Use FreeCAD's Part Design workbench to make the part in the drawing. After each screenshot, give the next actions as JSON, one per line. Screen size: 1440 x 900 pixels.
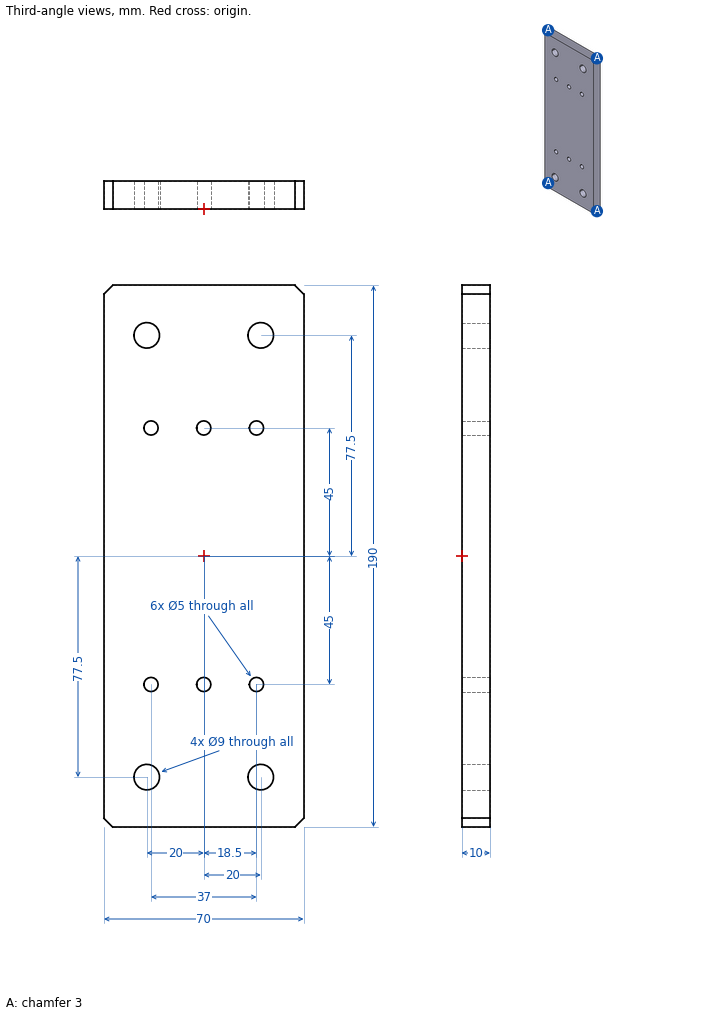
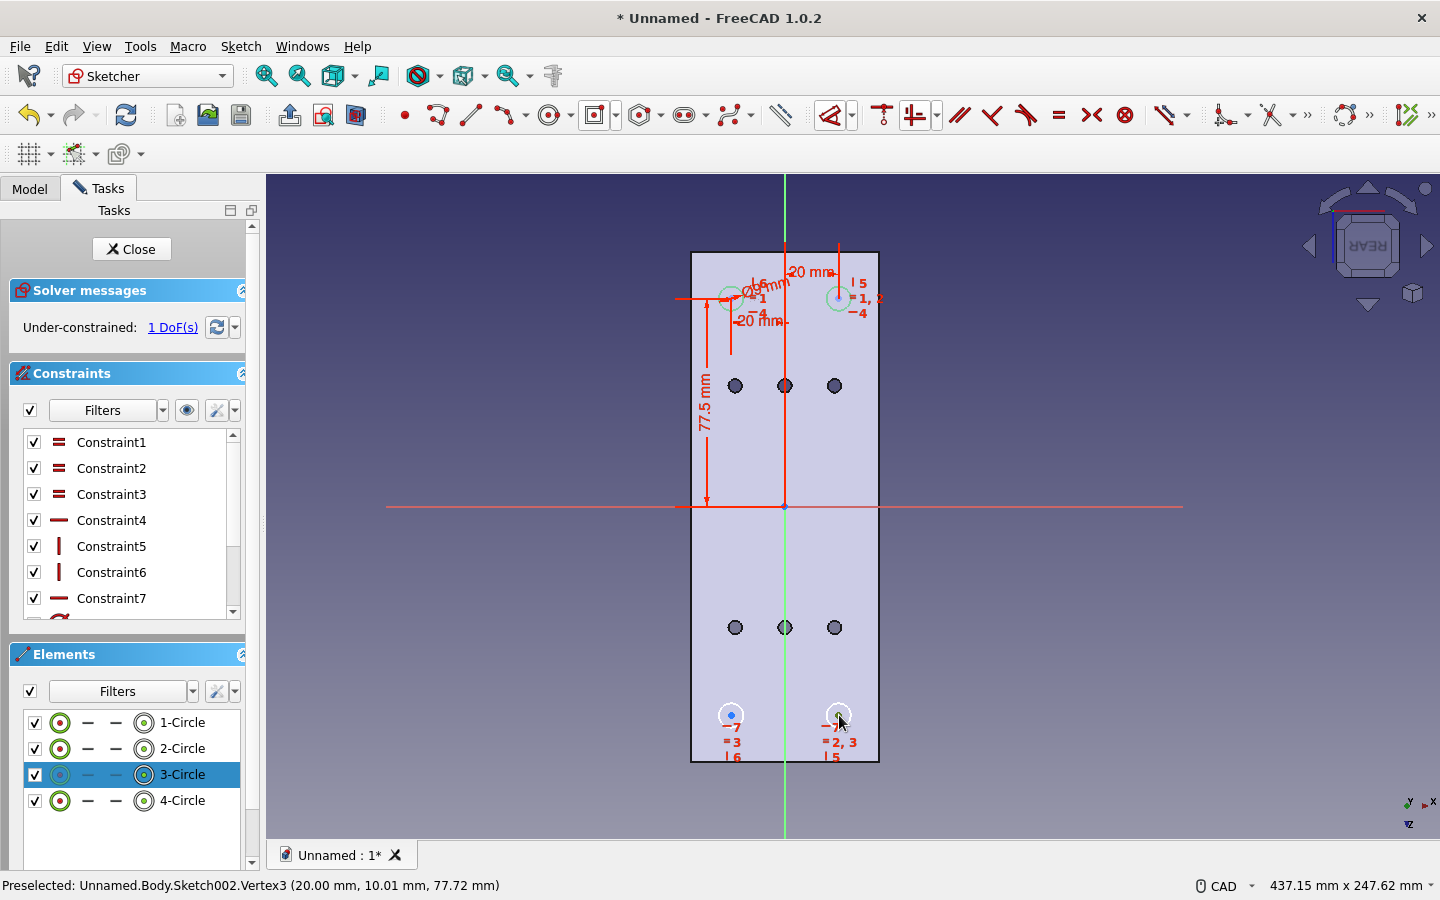
{"action": "left_click", "coordinate": [852, 116]}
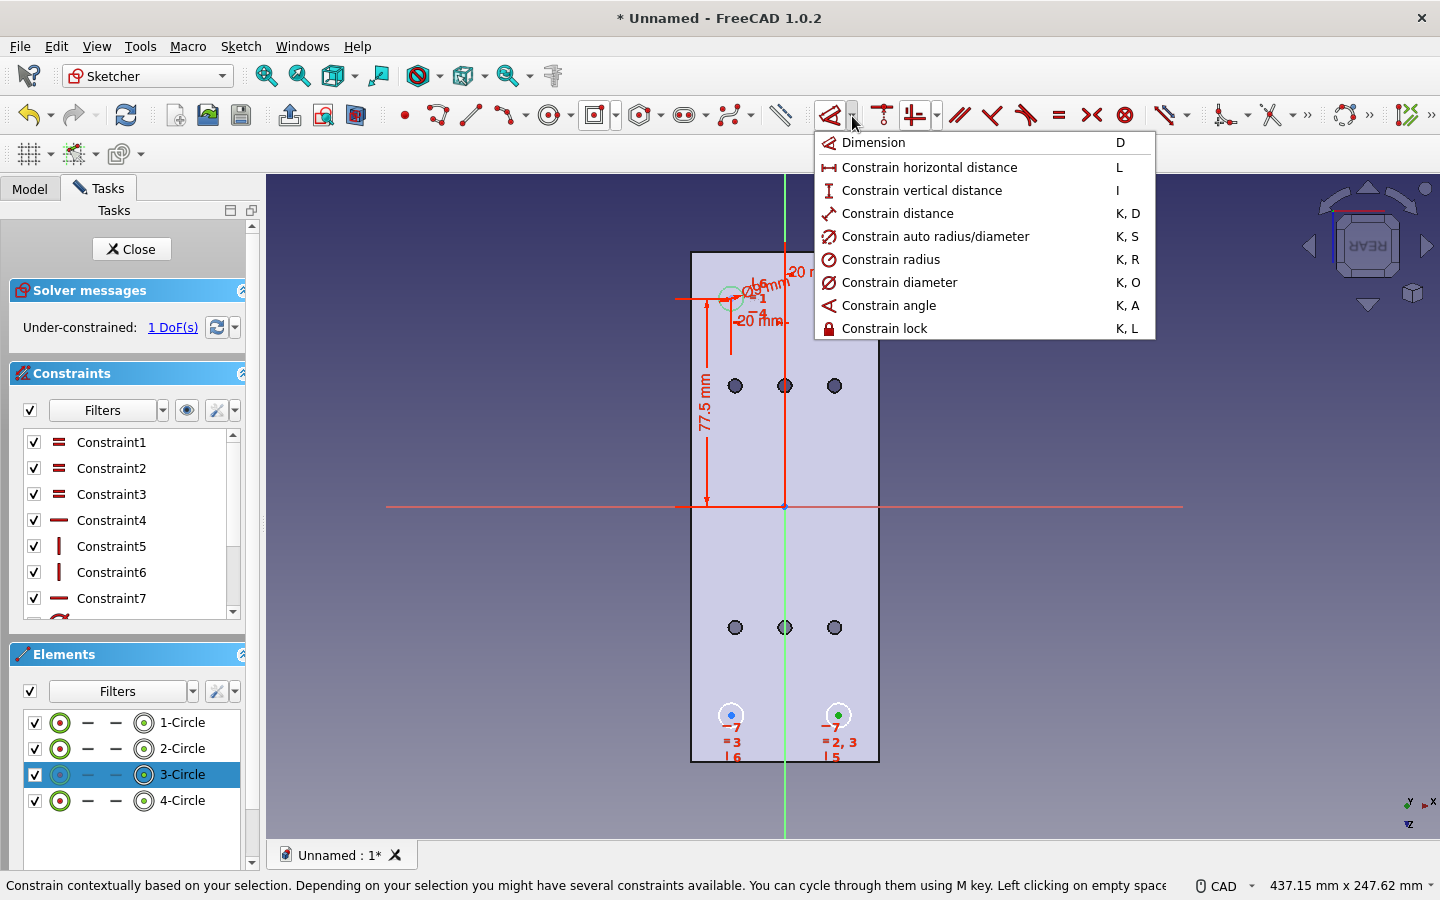
{"action": "left_click", "coordinate": [985, 190]}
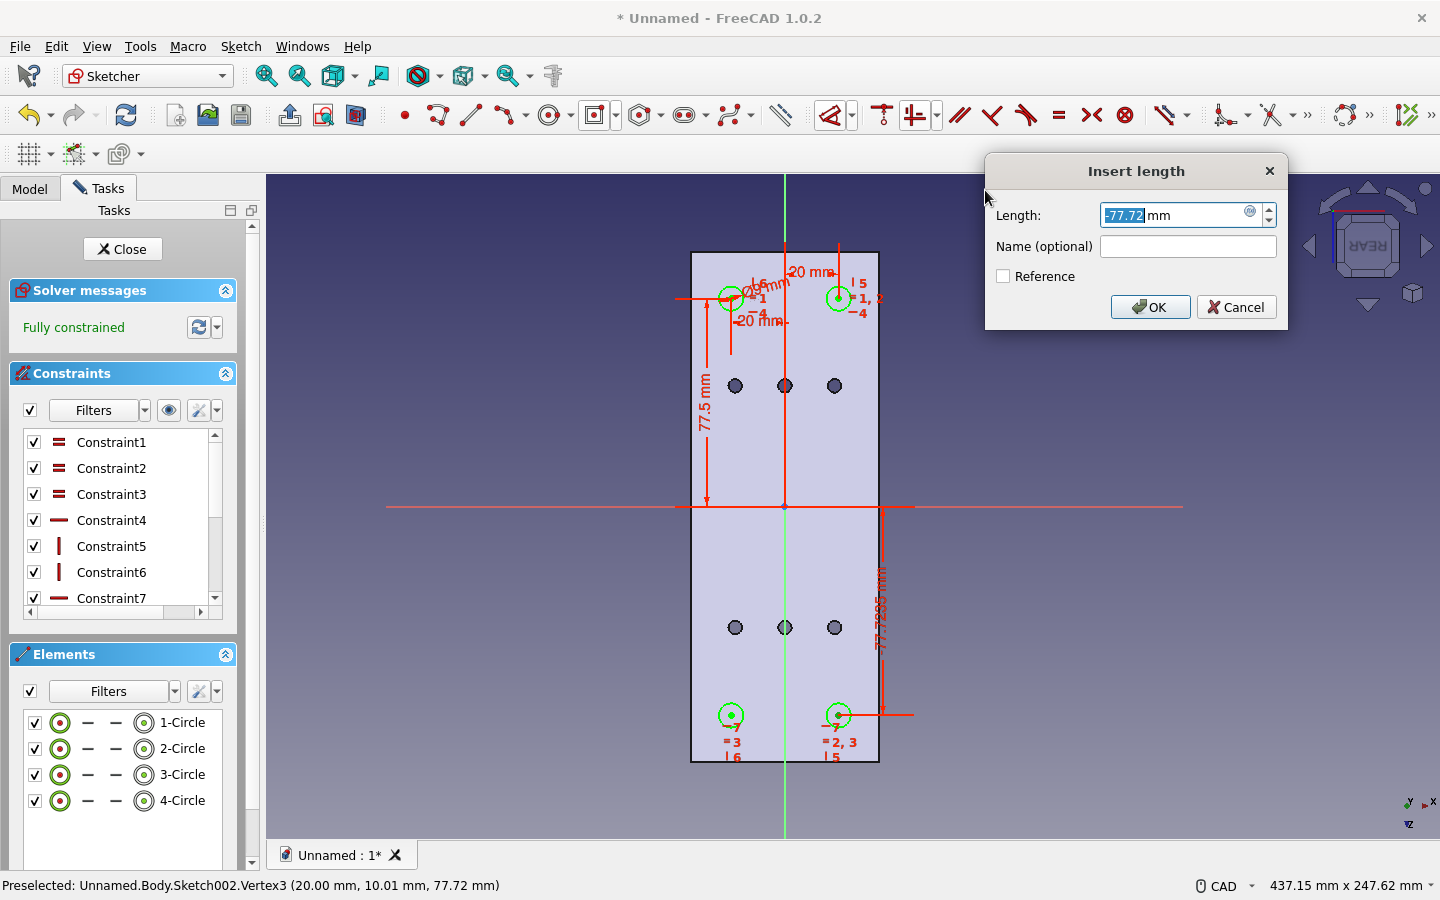
{"action": "type", "text": "-77.5"}
{"action": "key", "text": "Return"}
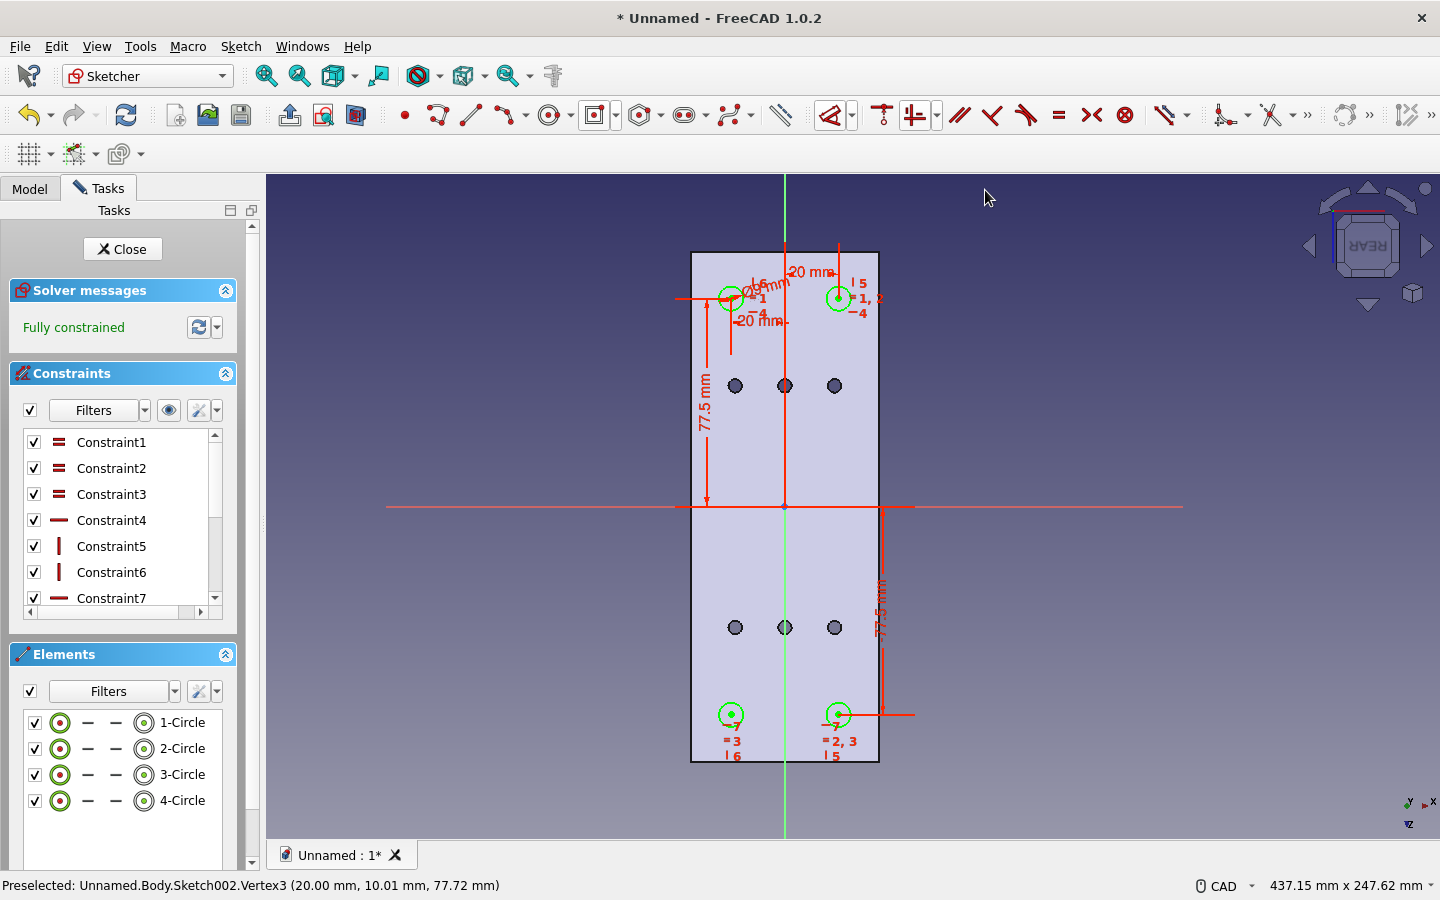
{"action": "left_click", "coordinate": [123, 249]}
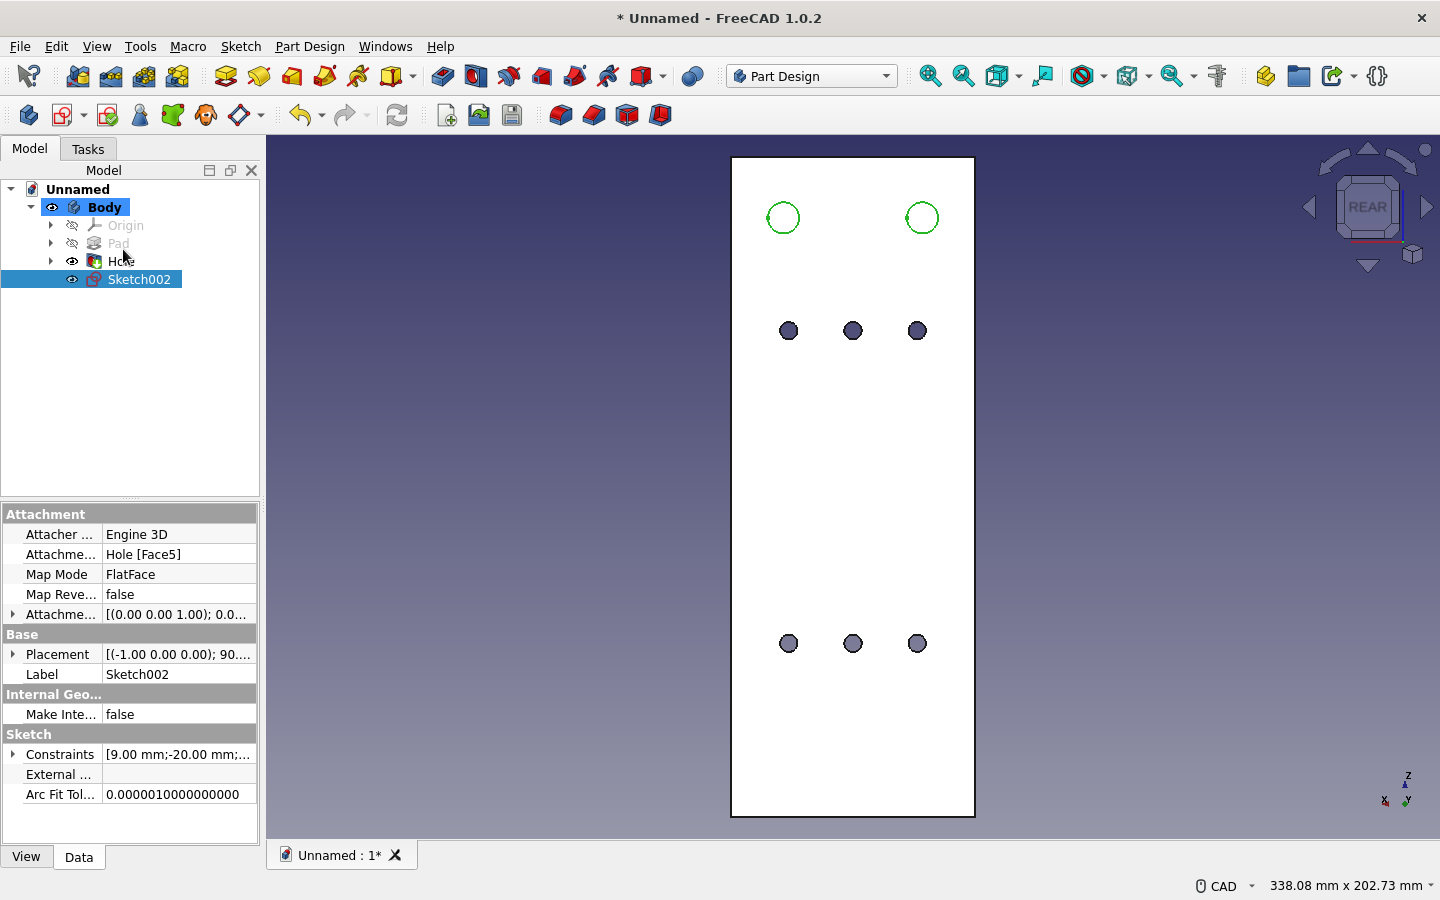
{"action": "left_click", "coordinate": [476, 76]}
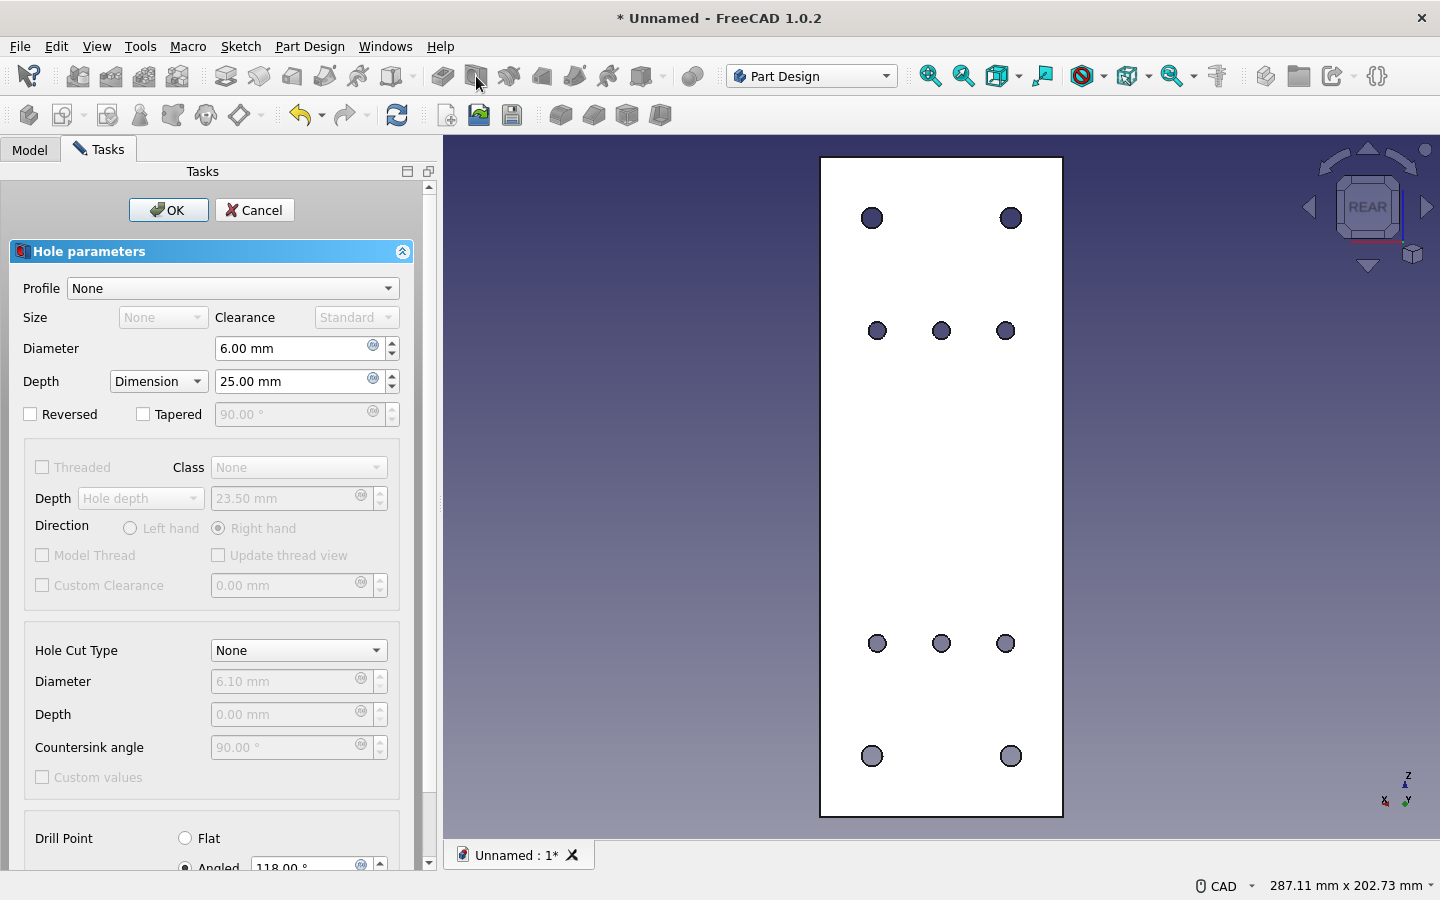
{"action": "triple_click", "coordinate": [300, 348]}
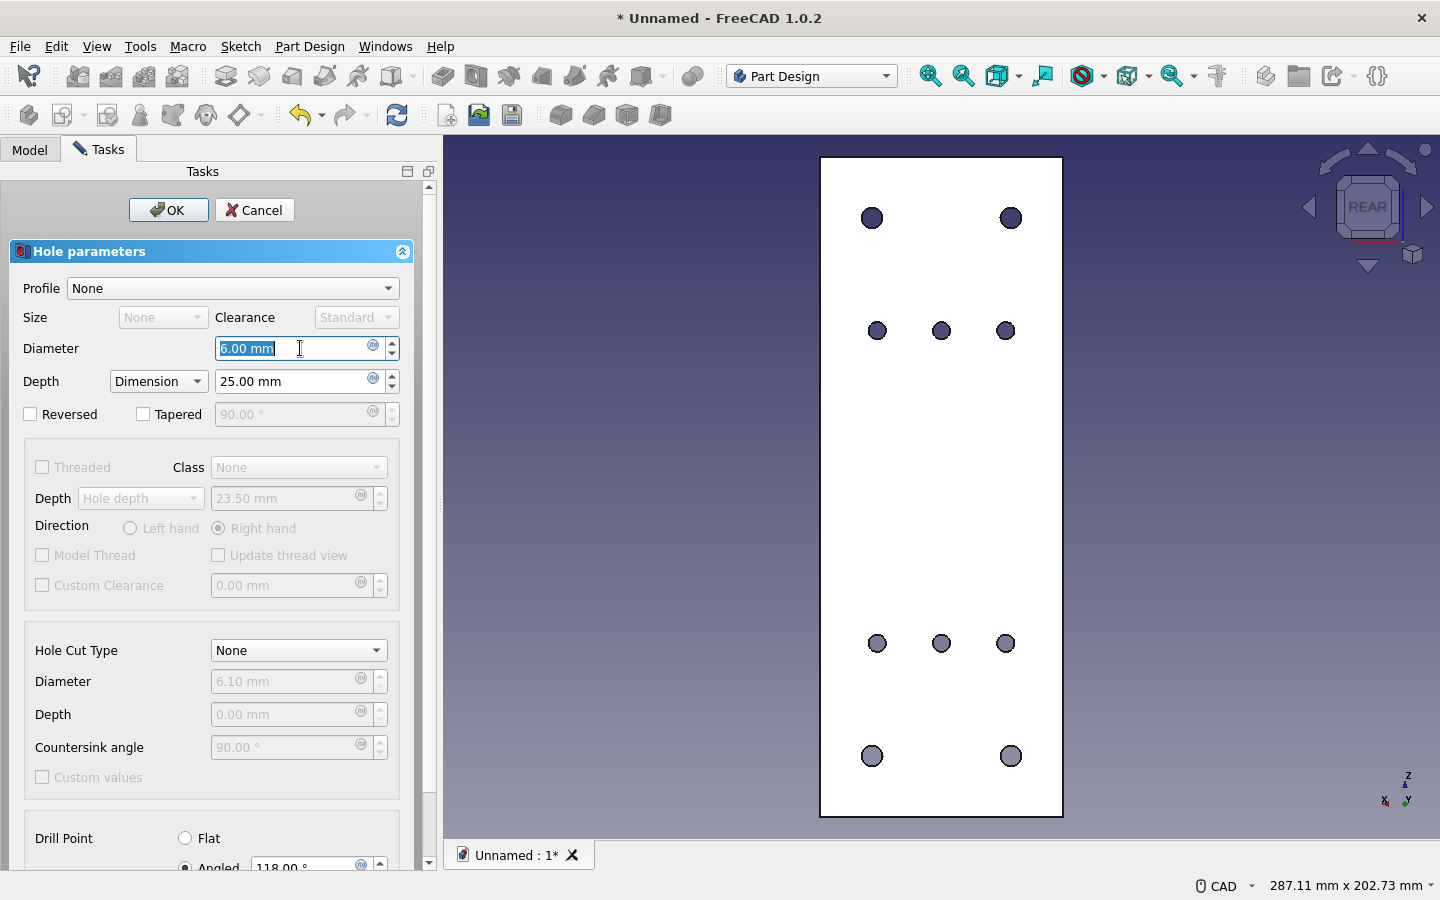
{"action": "type", "text": "9"}
{"action": "key", "text": "Tab"}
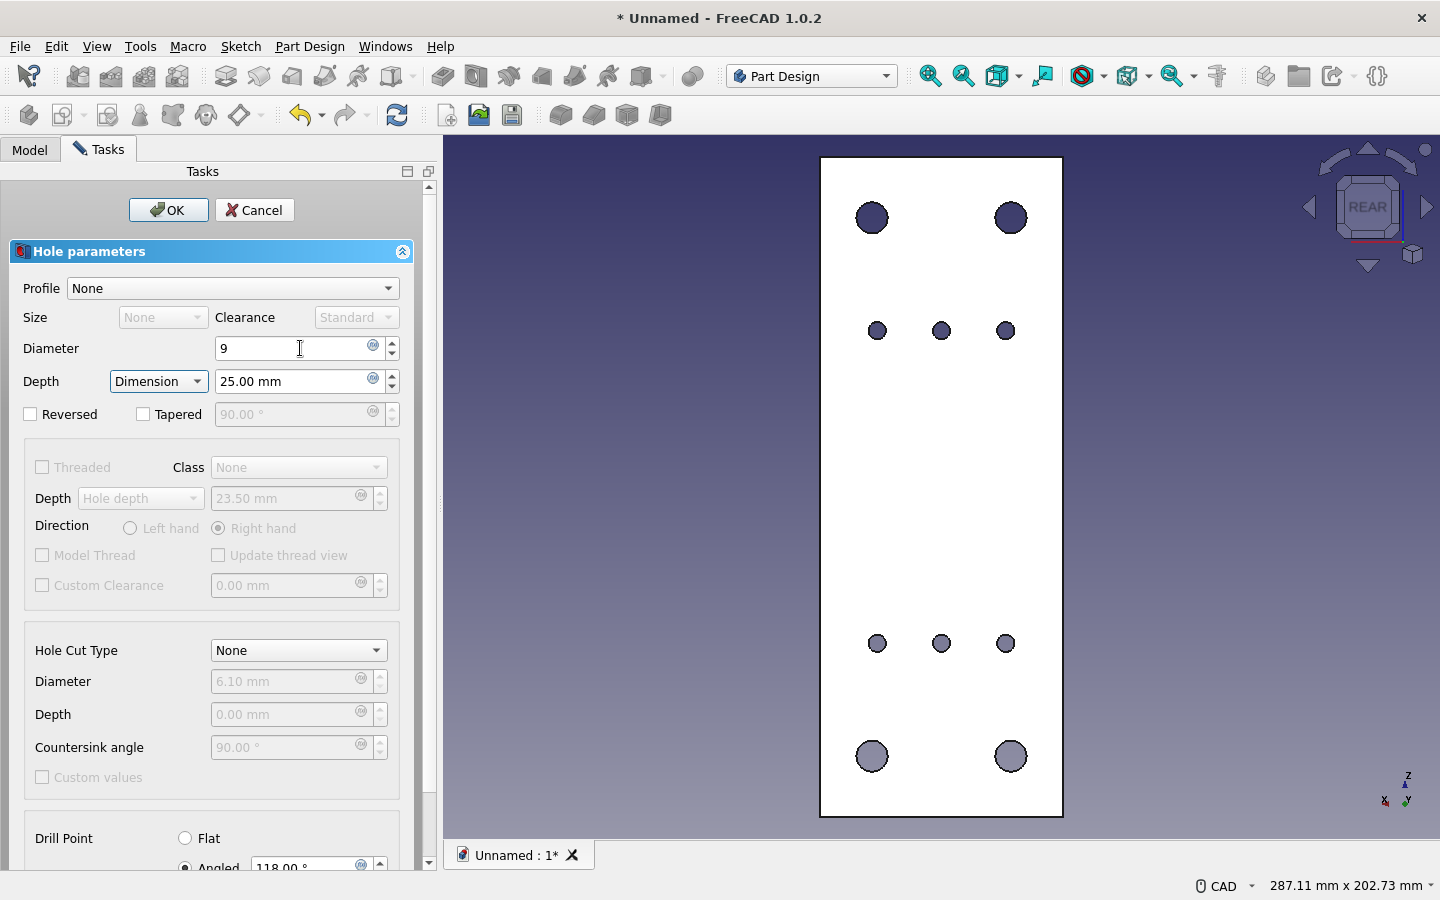
{"action": "left_click", "coordinate": [160, 382]}